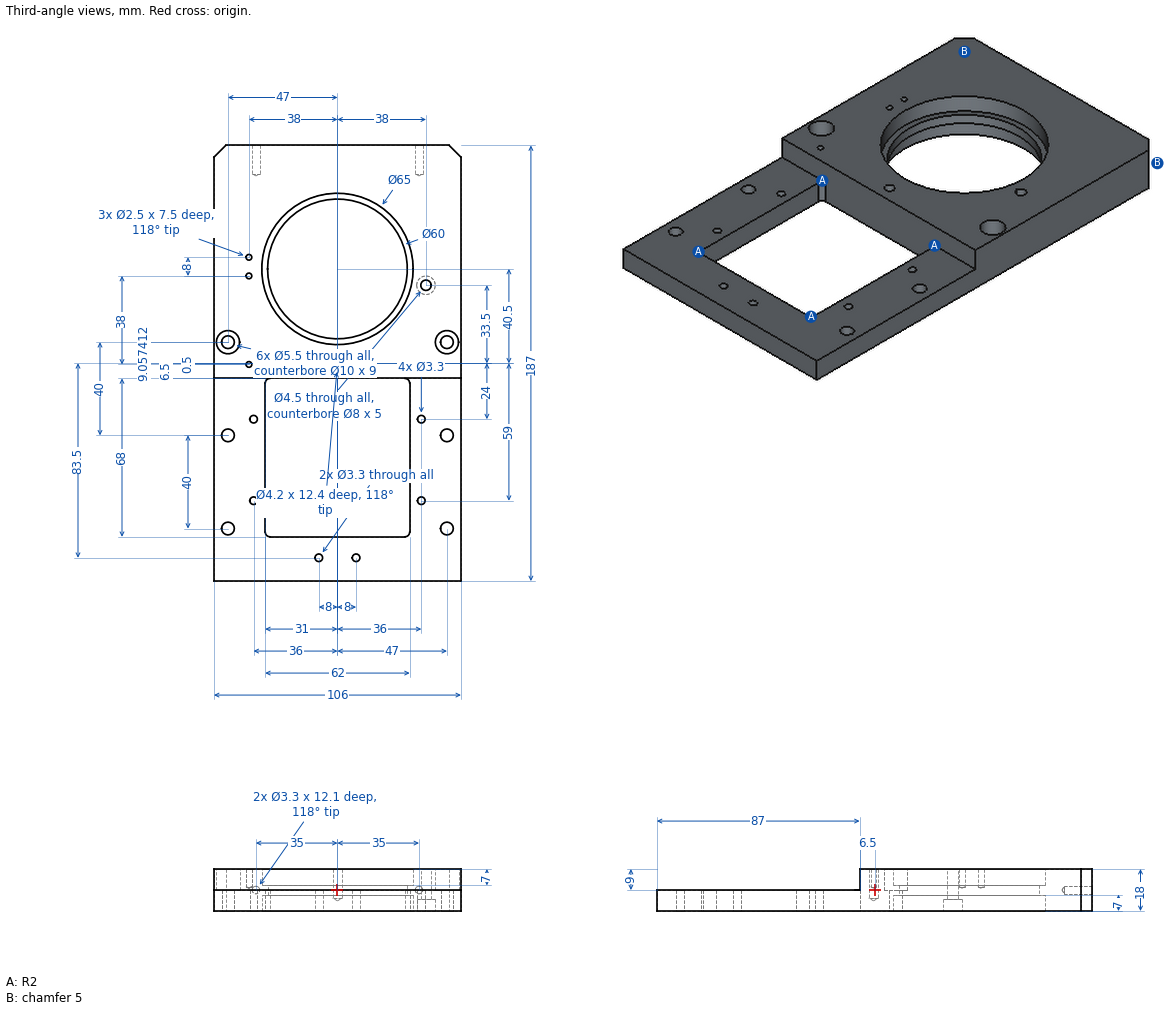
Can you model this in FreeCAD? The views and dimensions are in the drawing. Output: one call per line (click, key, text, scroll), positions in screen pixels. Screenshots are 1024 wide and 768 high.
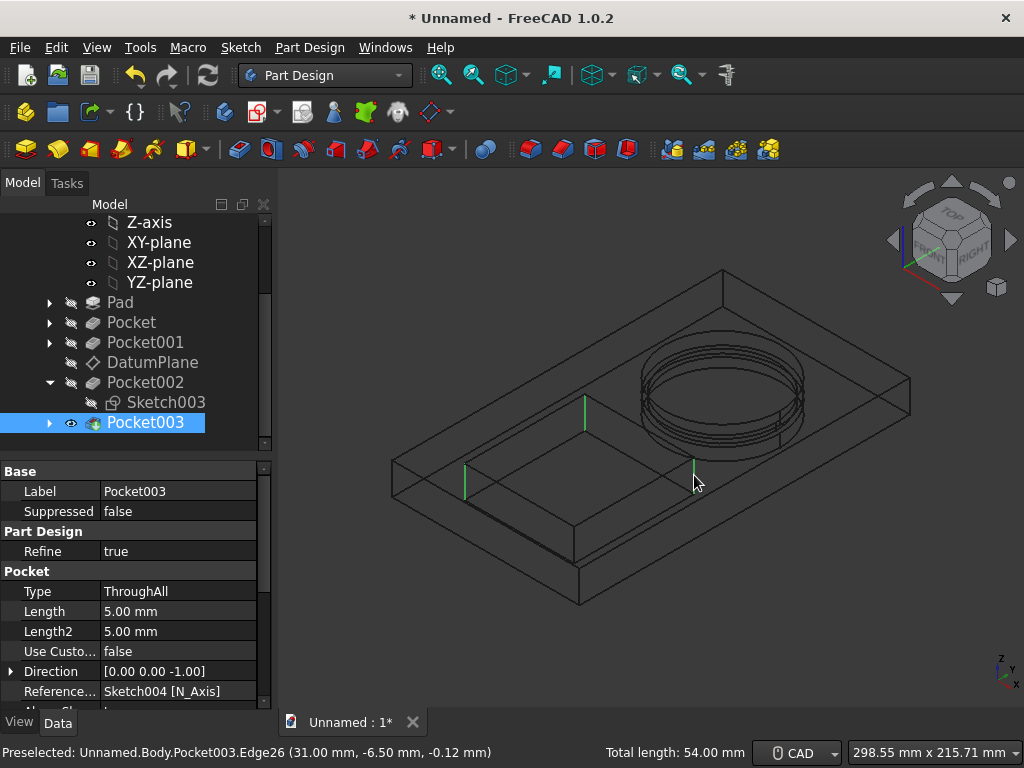
click(574, 544, ctrl)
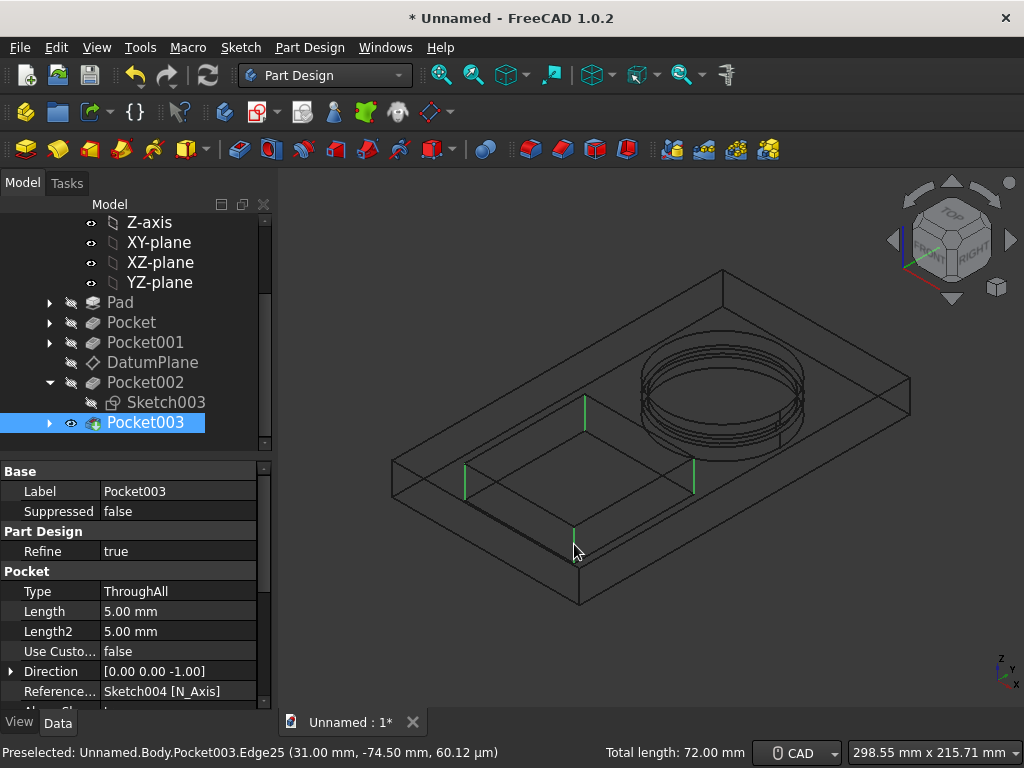
key(v)
key(1)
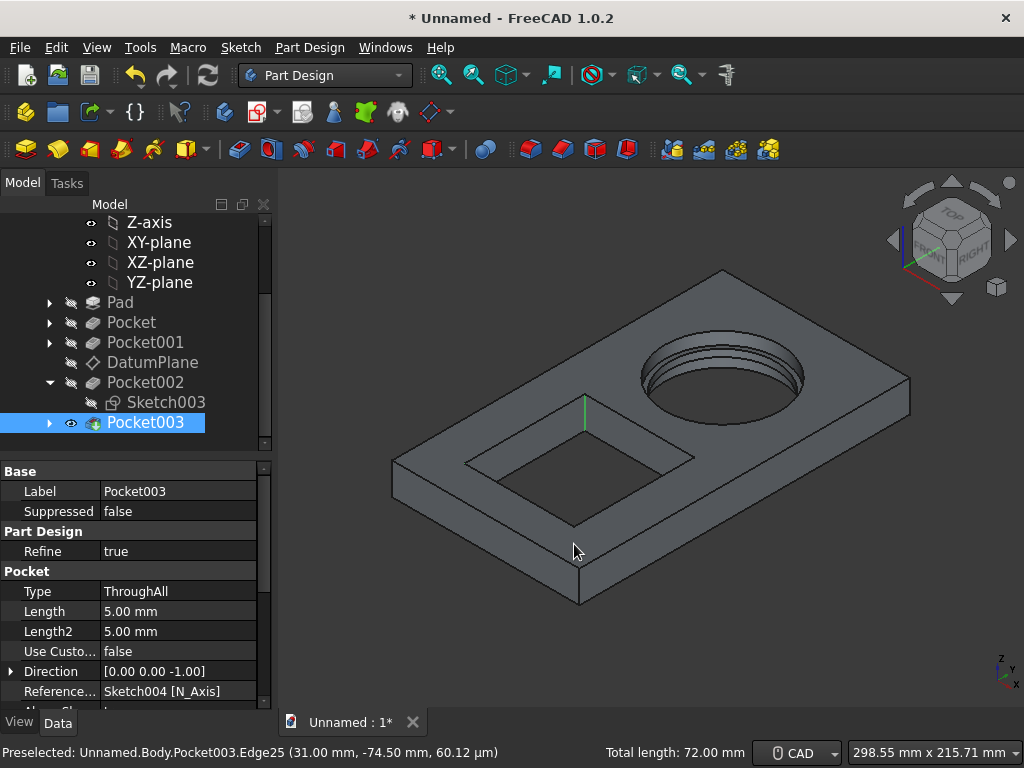
click(532, 150)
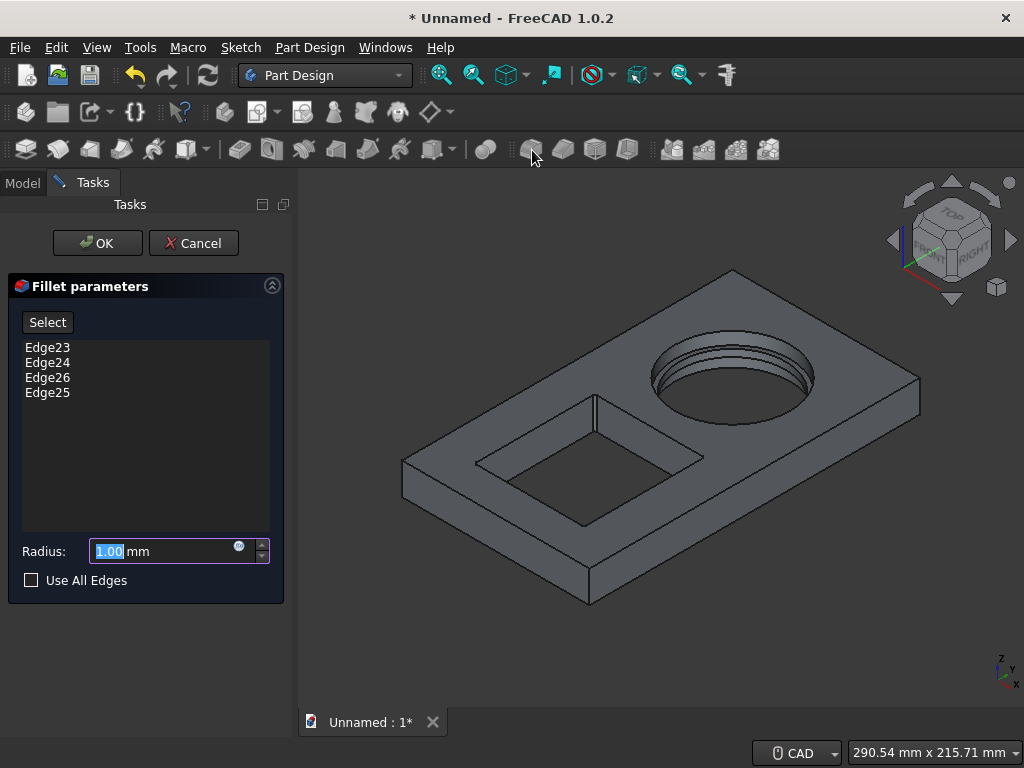
text(2)
key(Tab)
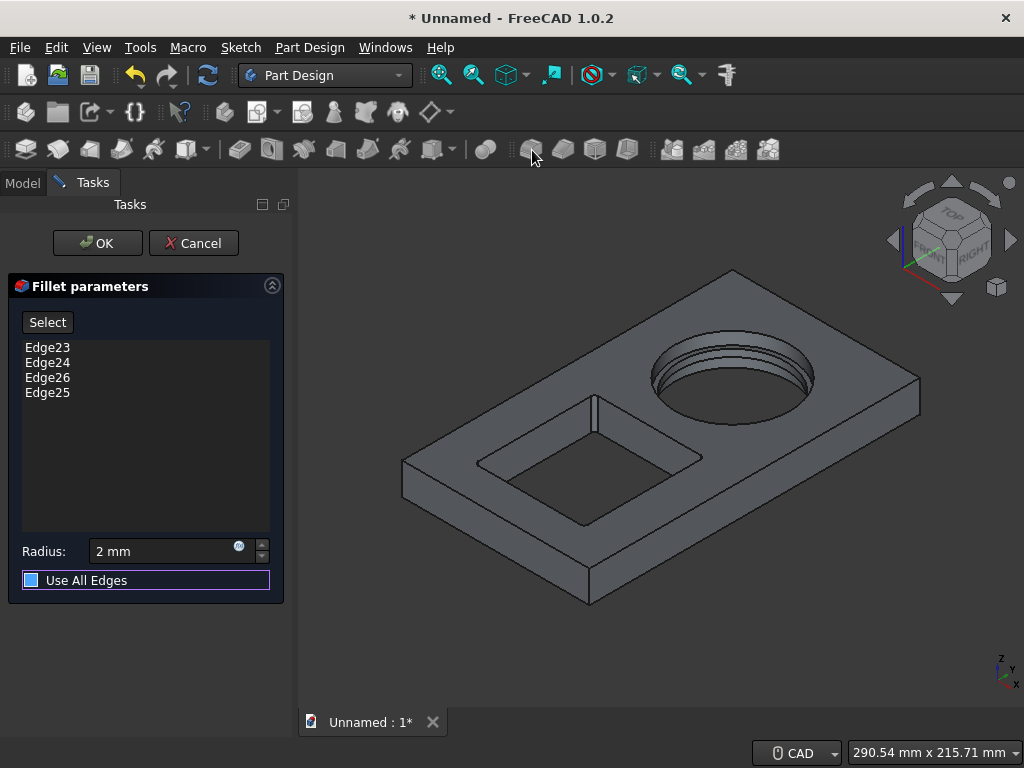
click(98, 243)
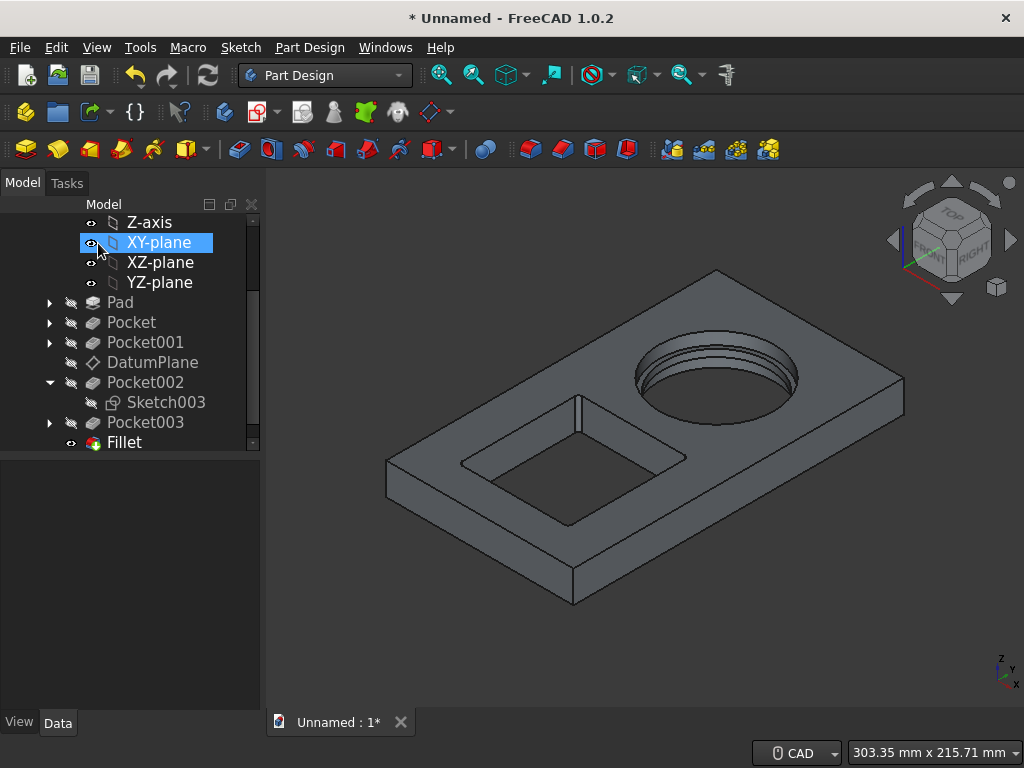
click(880, 409)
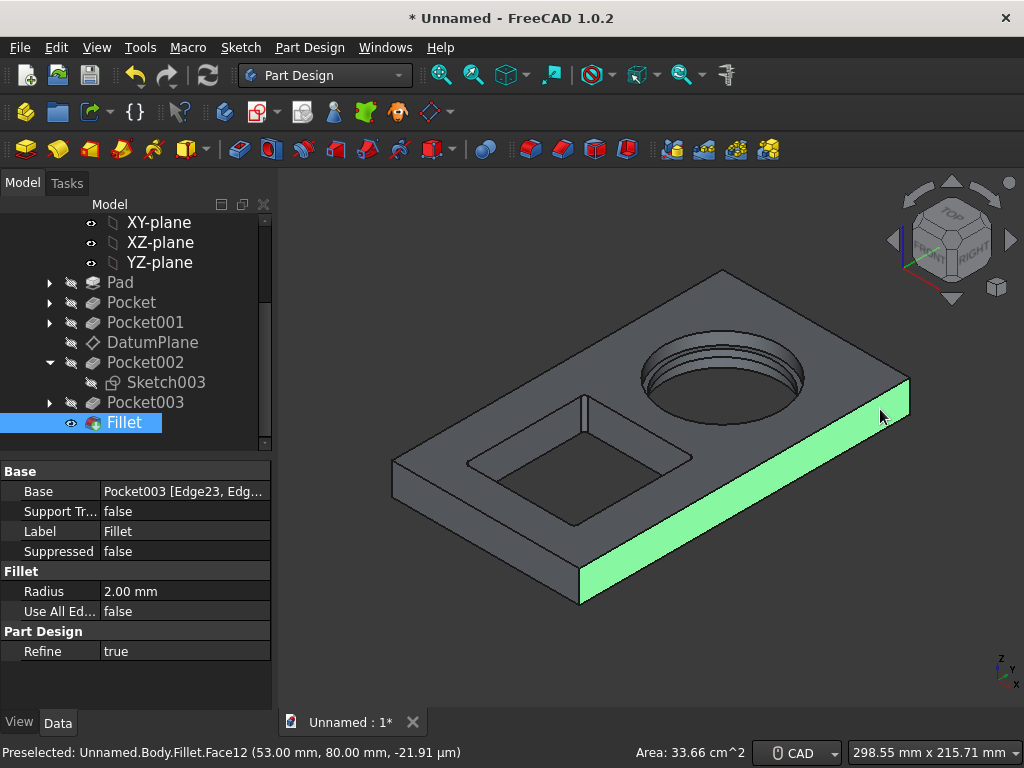
click(258, 112)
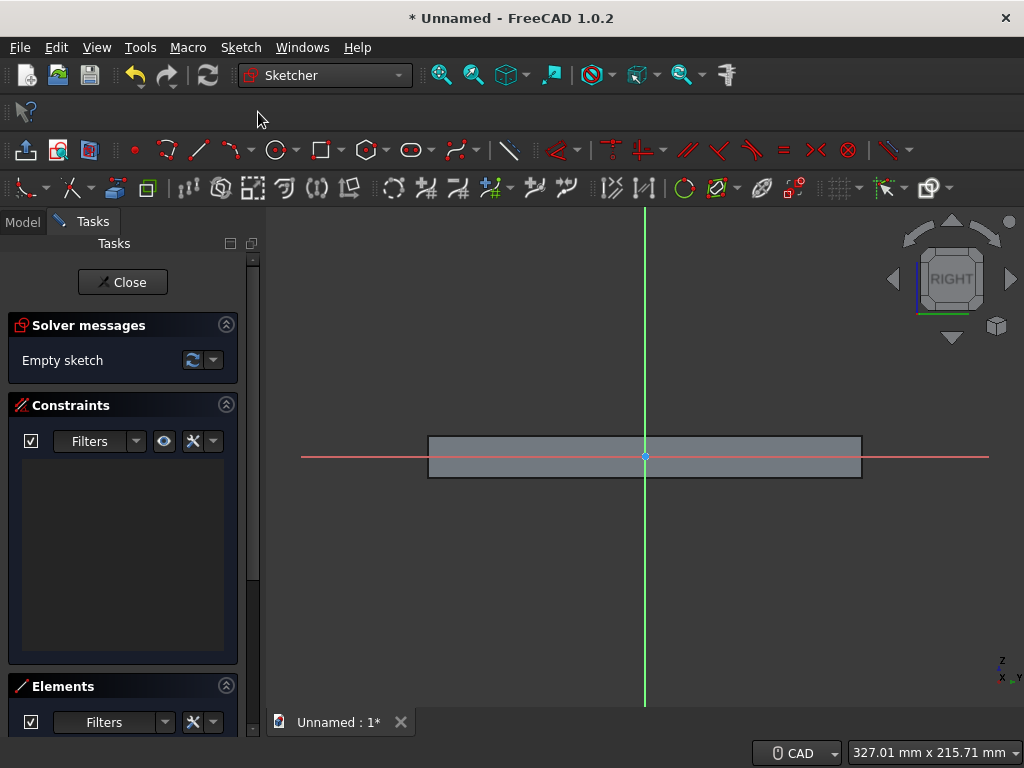
scroll(488, 434, up, 3)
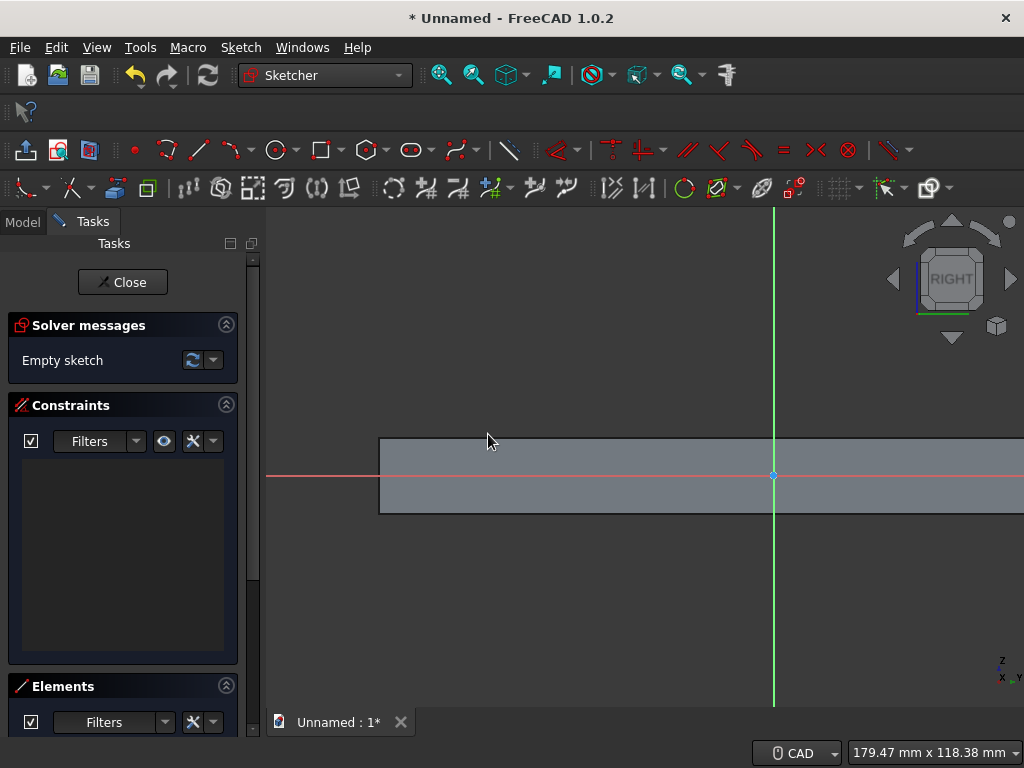
click(322, 150)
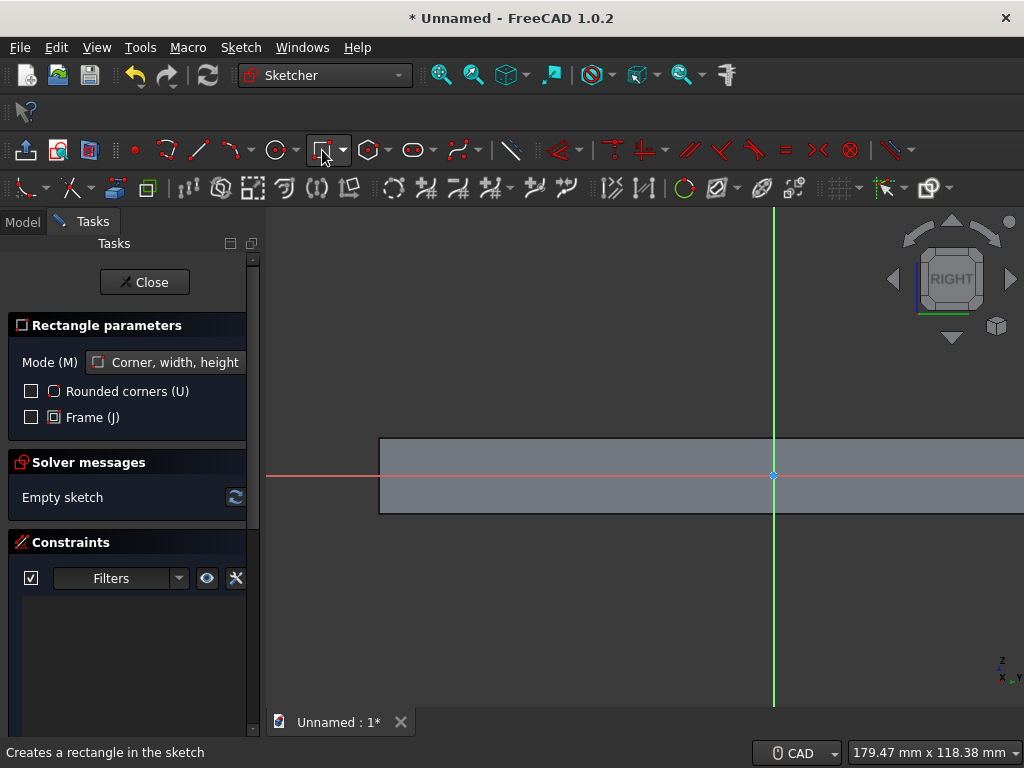
click(379, 438)
click(746, 476)
key(Escape)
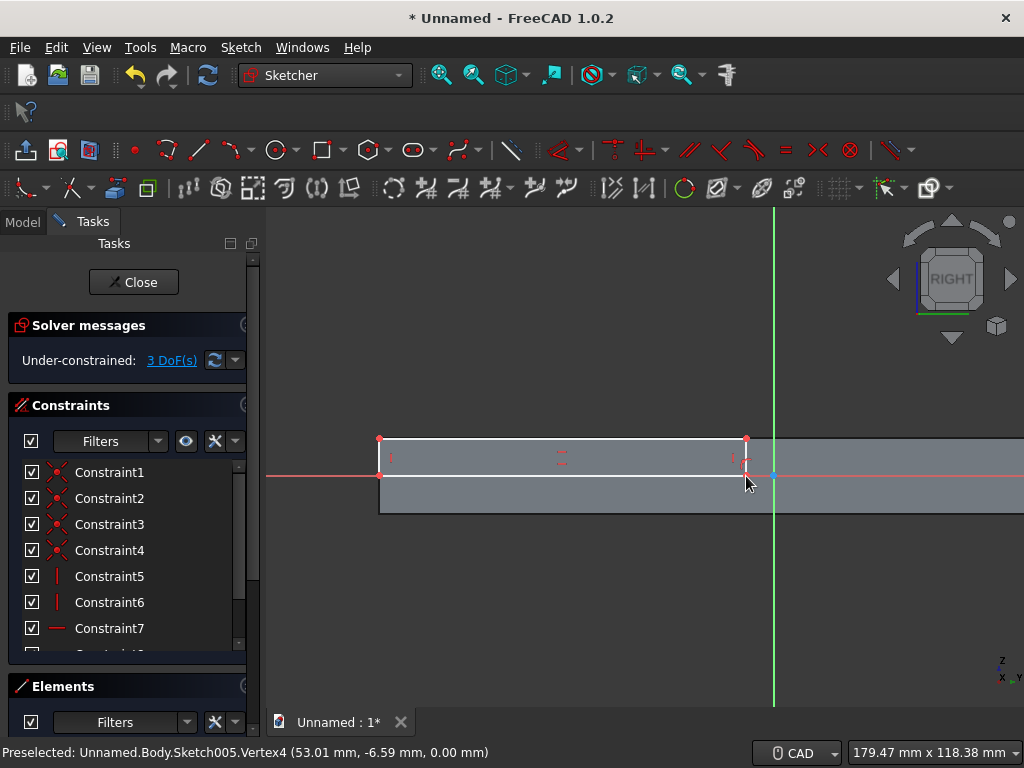
click(558, 150)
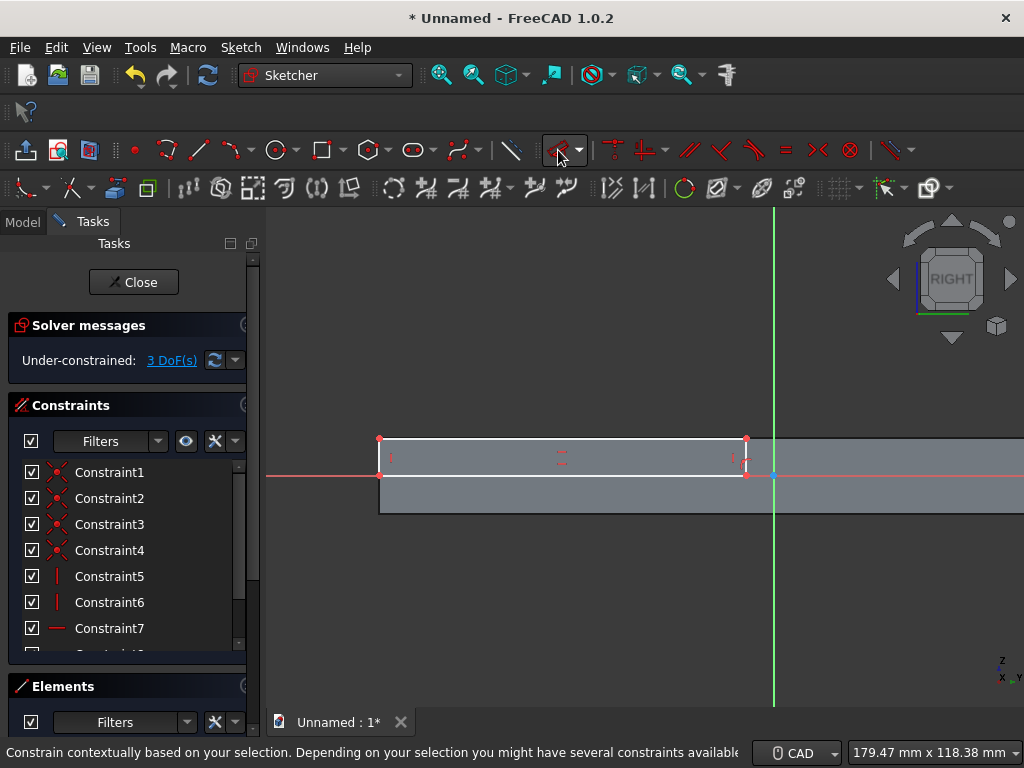
scroll(379, 450, up, 2)